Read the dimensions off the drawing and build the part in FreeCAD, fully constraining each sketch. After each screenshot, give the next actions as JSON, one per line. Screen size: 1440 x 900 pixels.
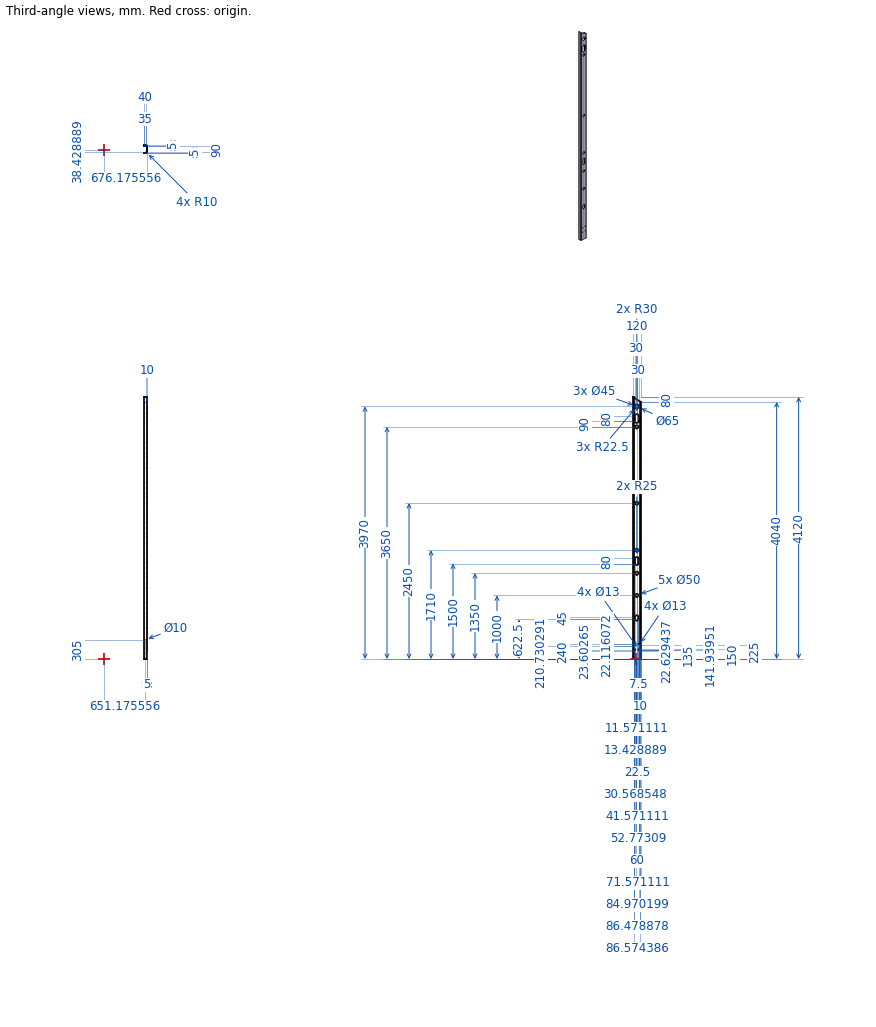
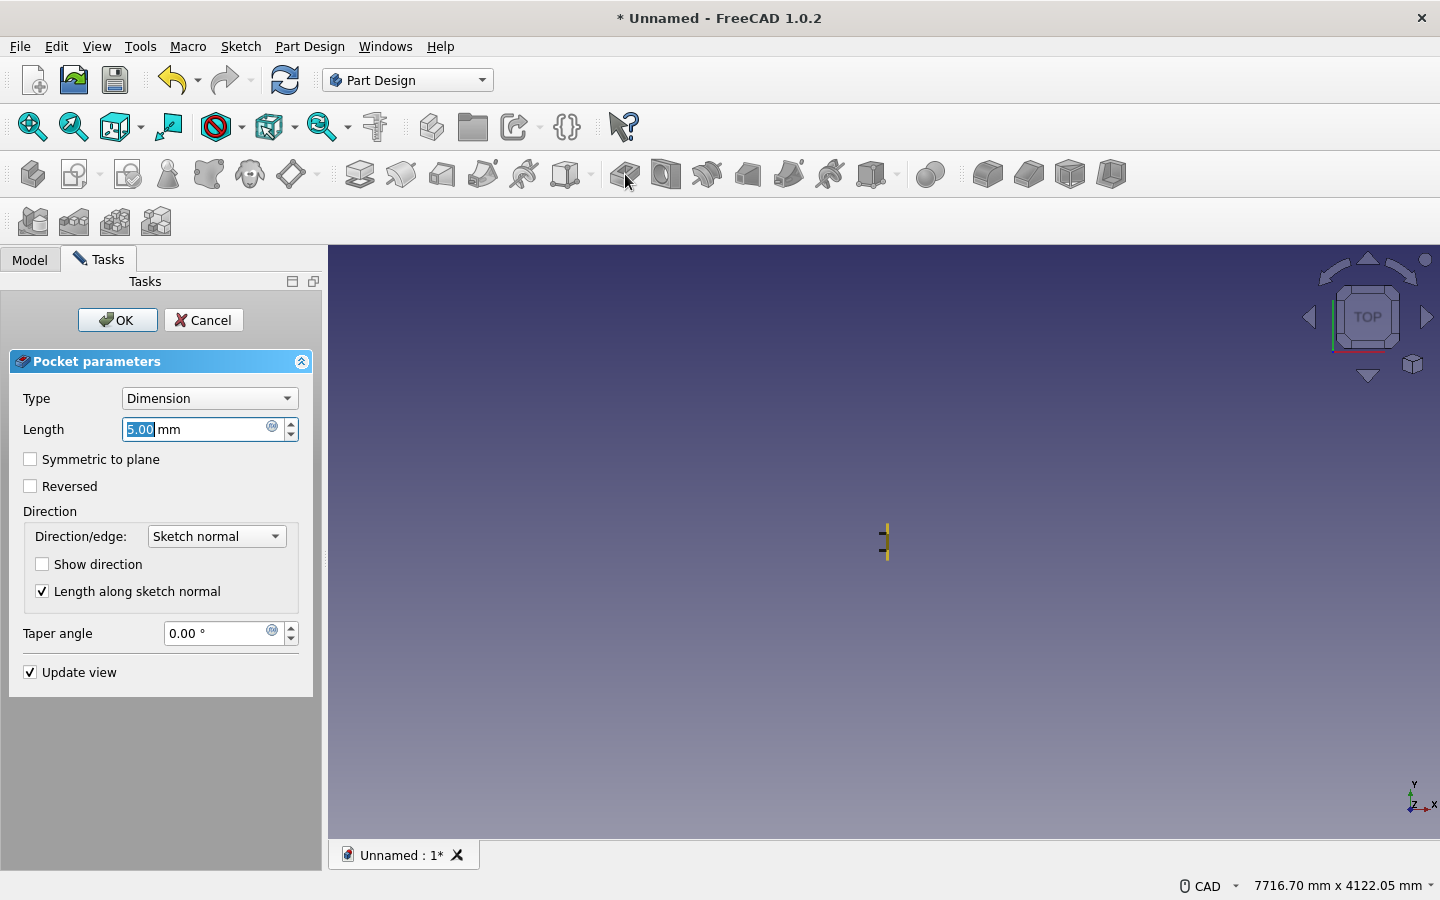
{"action": "type", "text": "10"}
{"action": "key", "text": "Tab"}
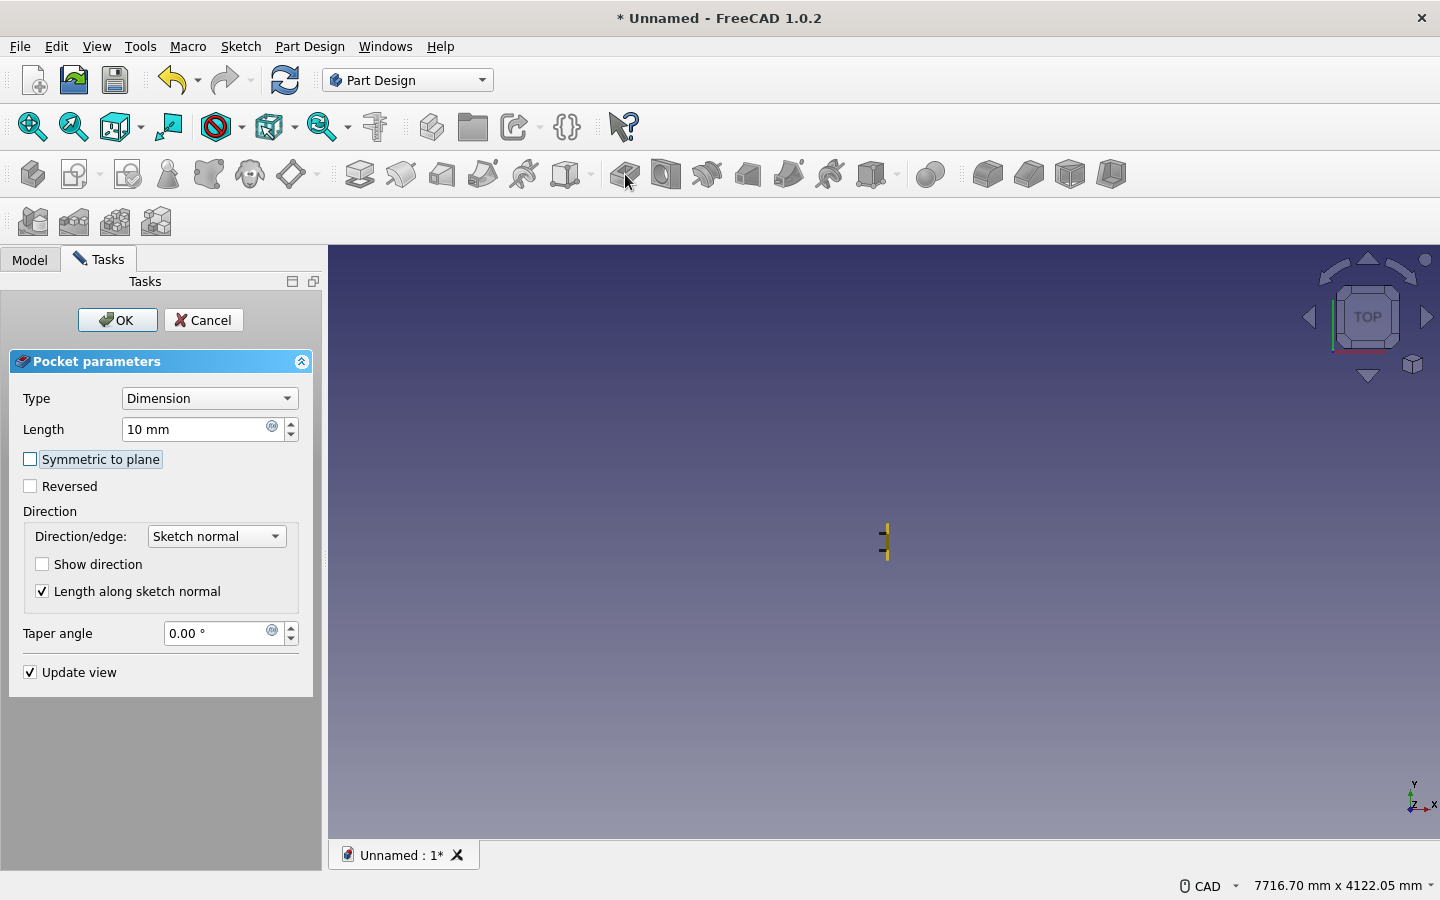
{"action": "left_click", "coordinate": [118, 320]}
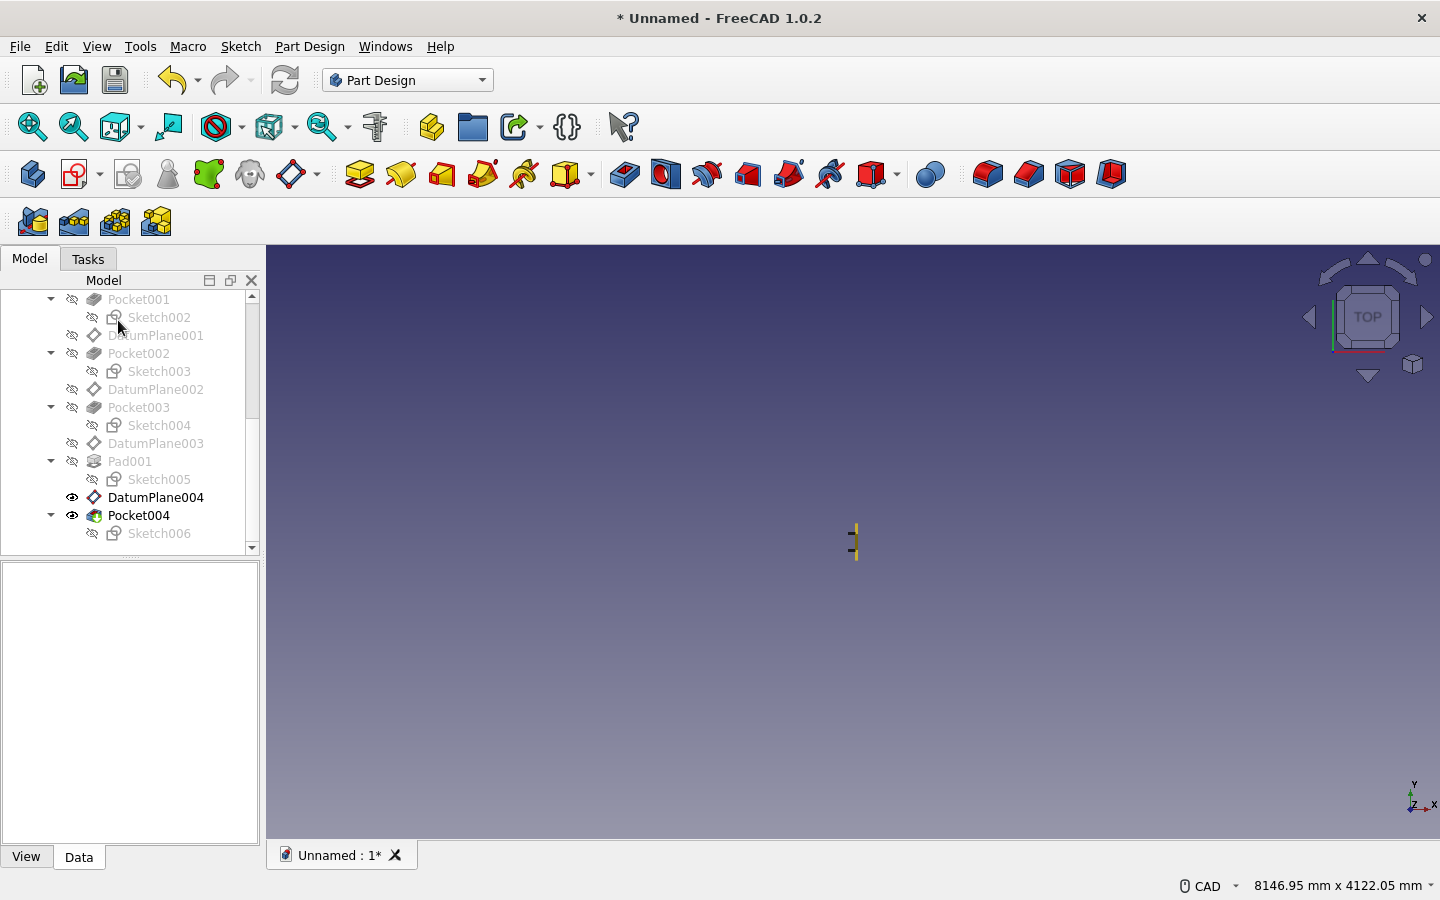
{"action": "left_click", "coordinate": [117, 497]}
{"action": "key", "text": "space"}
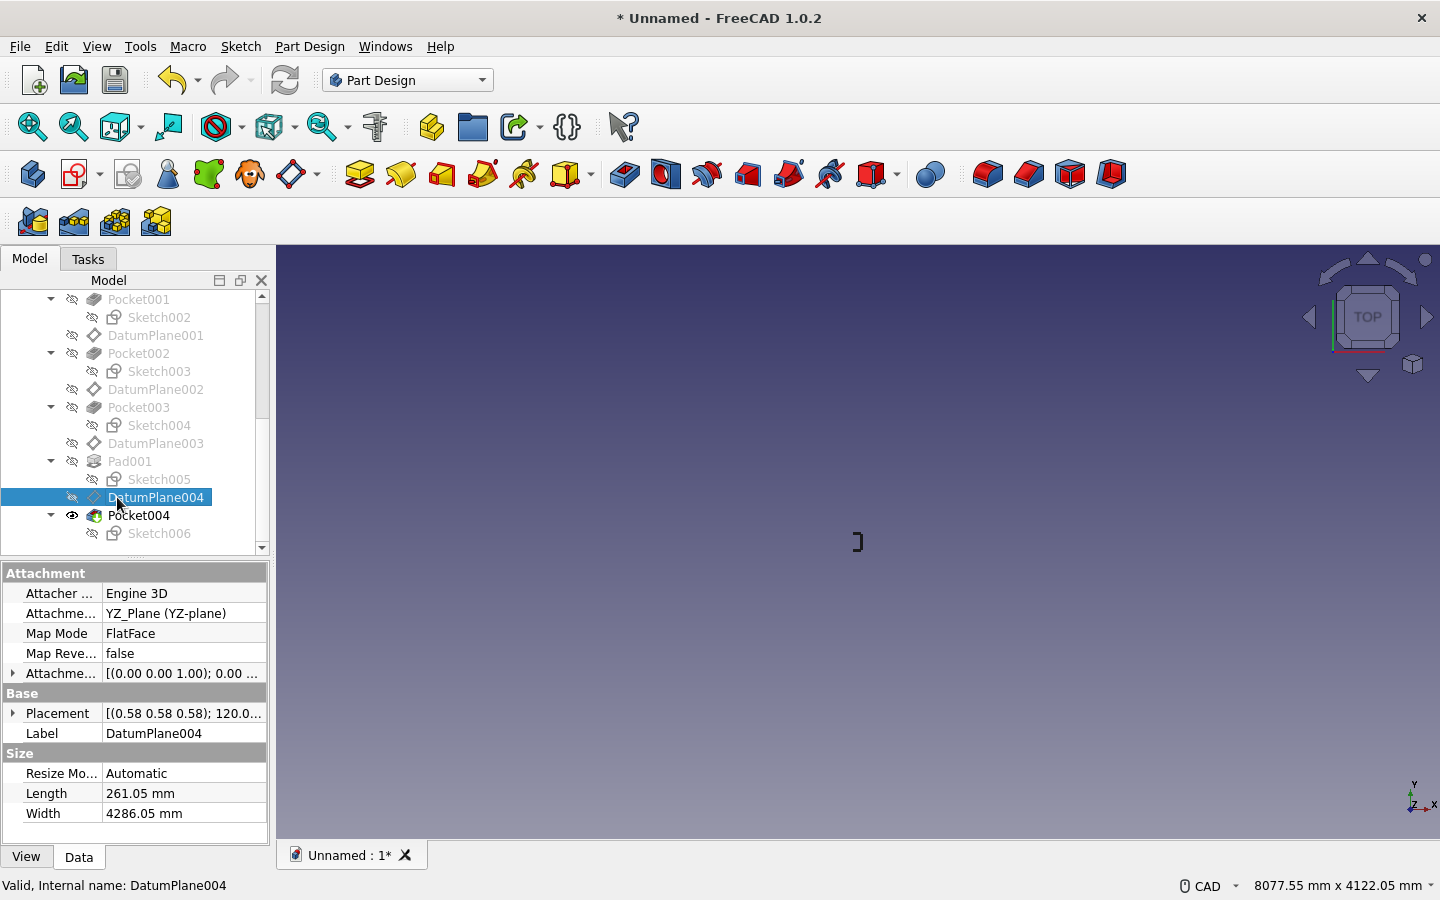
{"action": "key", "text": "v f"}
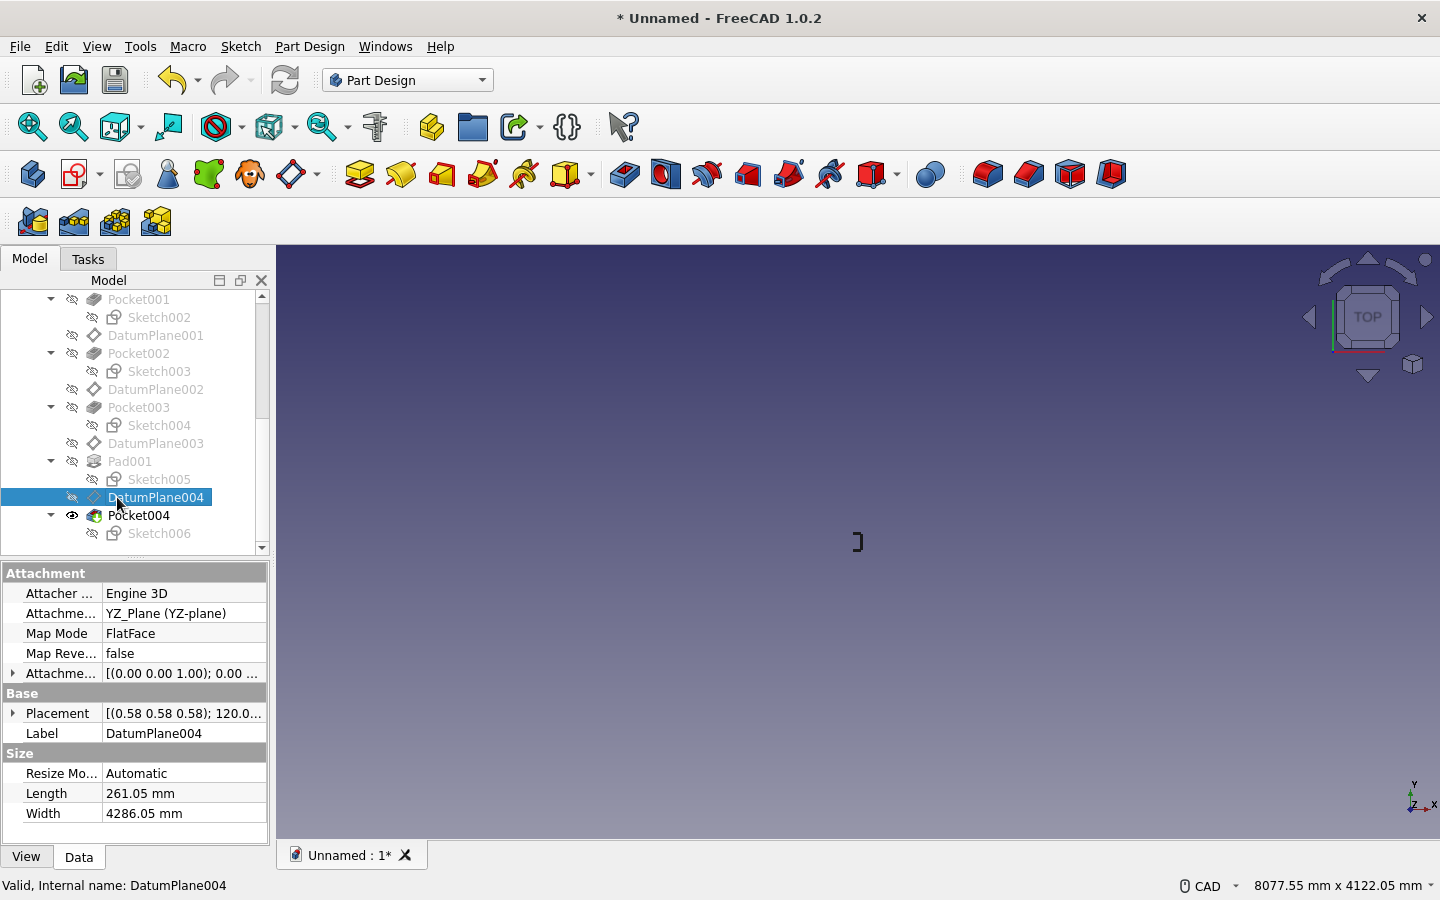
{"action": "key", "text": "0"}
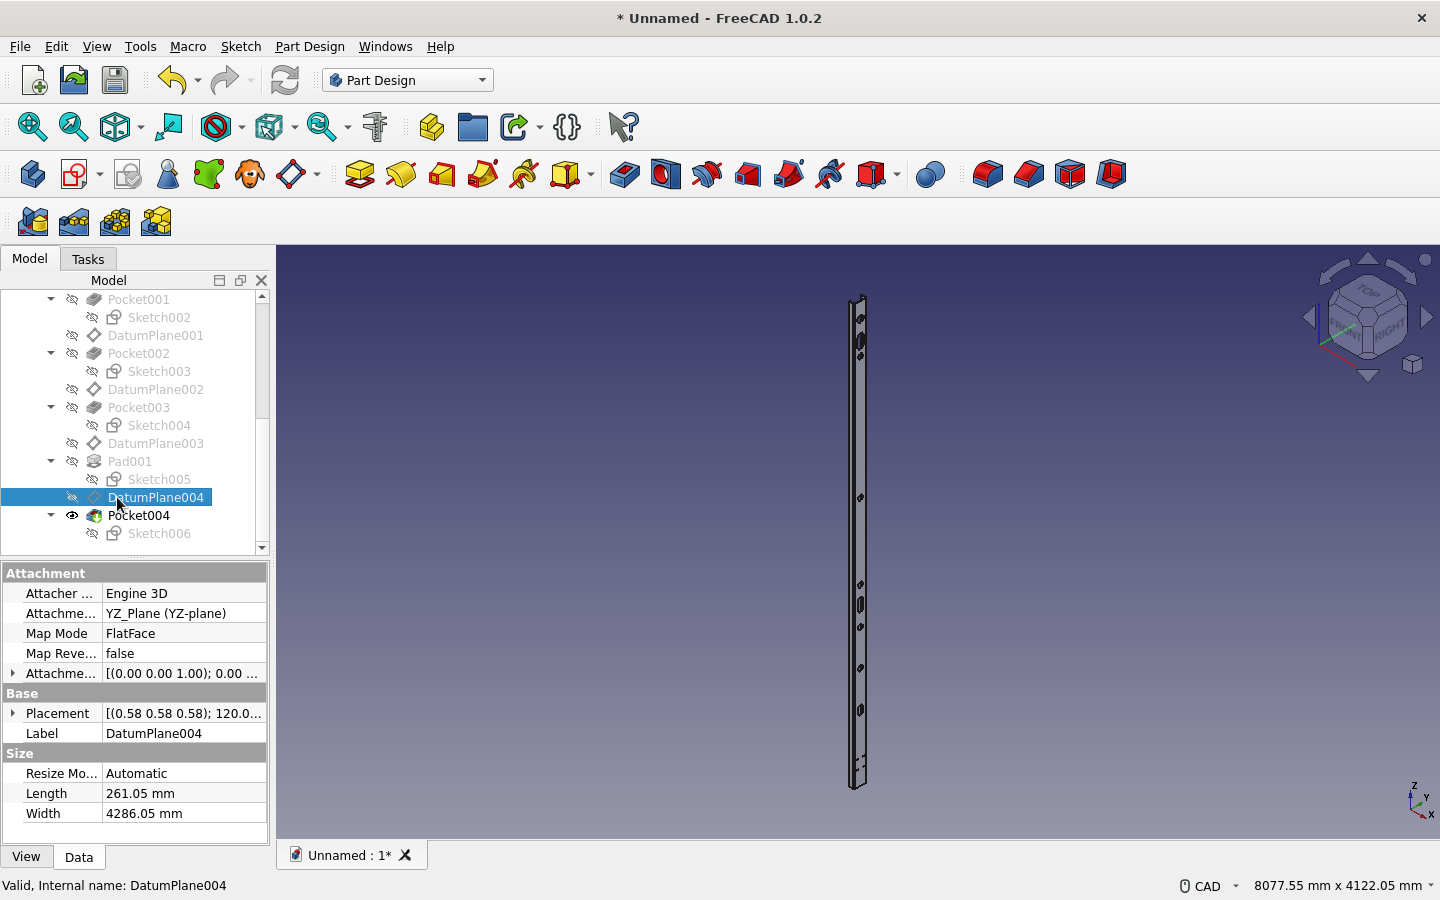
{"action": "key", "text": "3"}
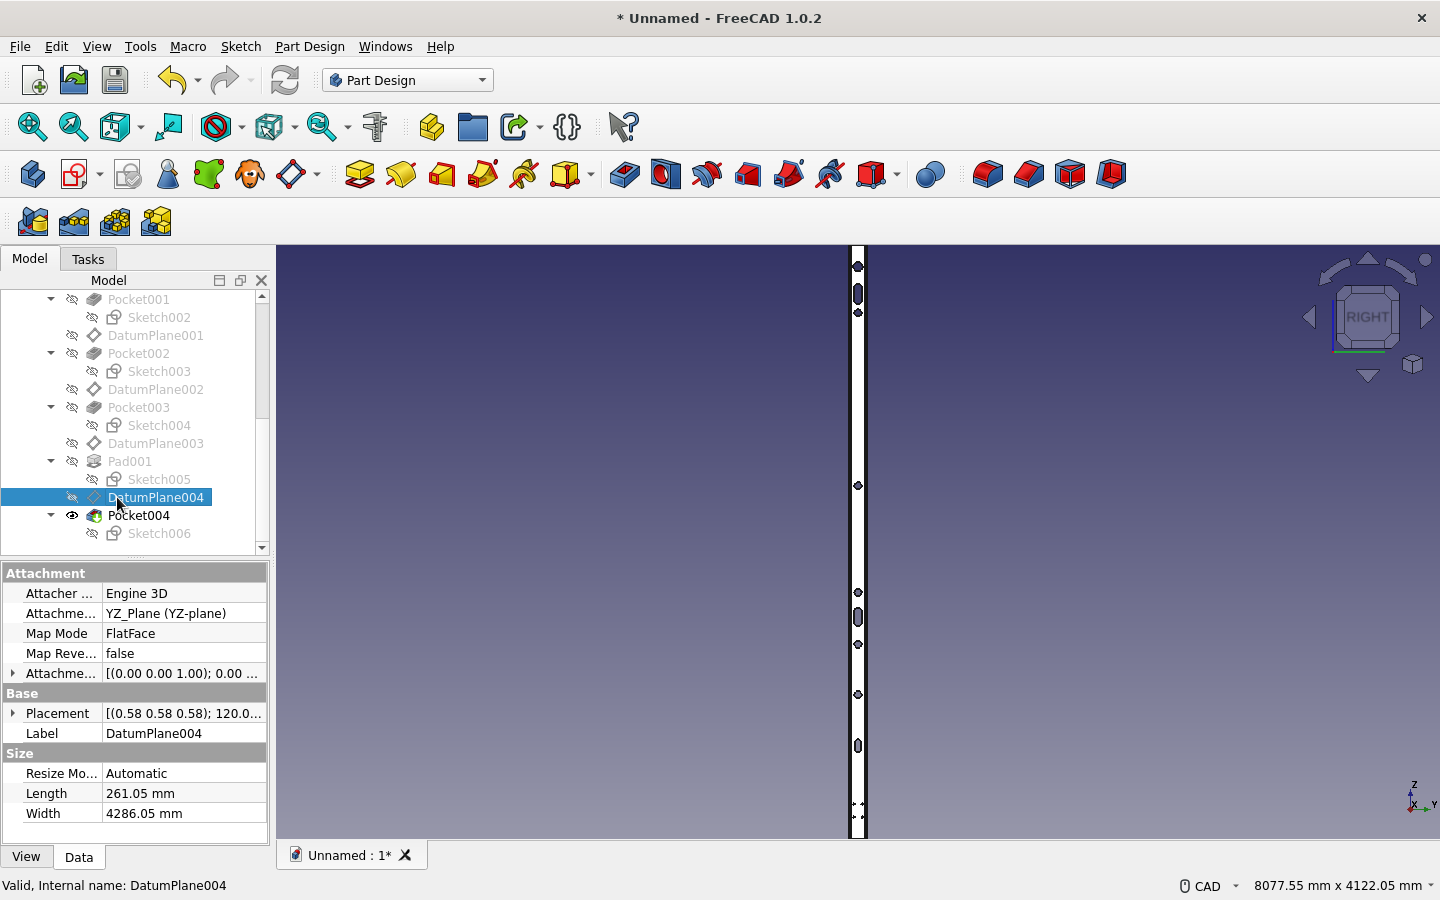
{"action": "key", "text": "v f"}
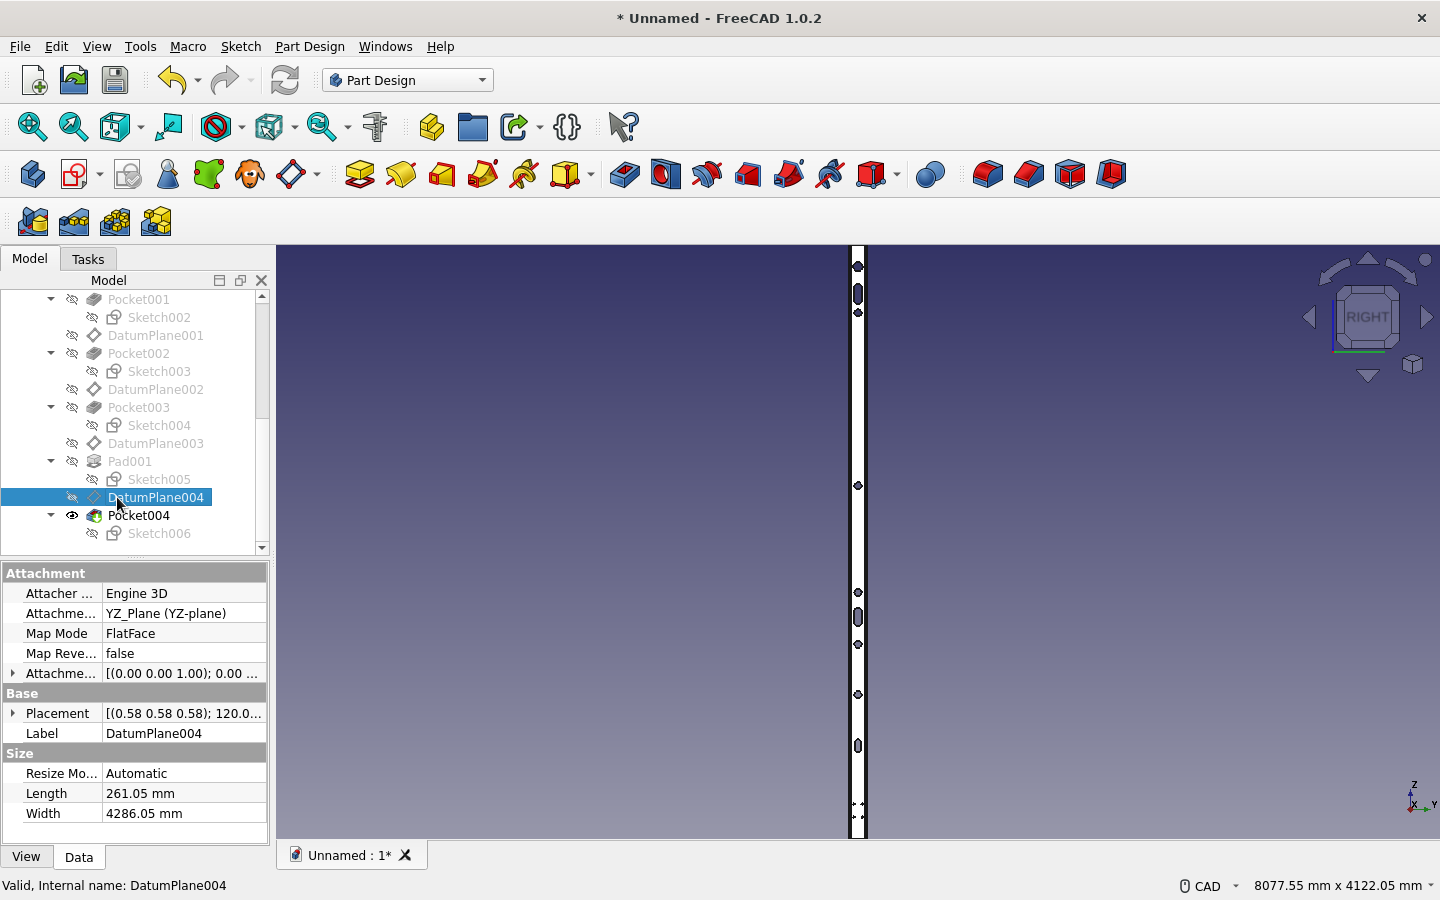
{"action": "key", "text": "2"}